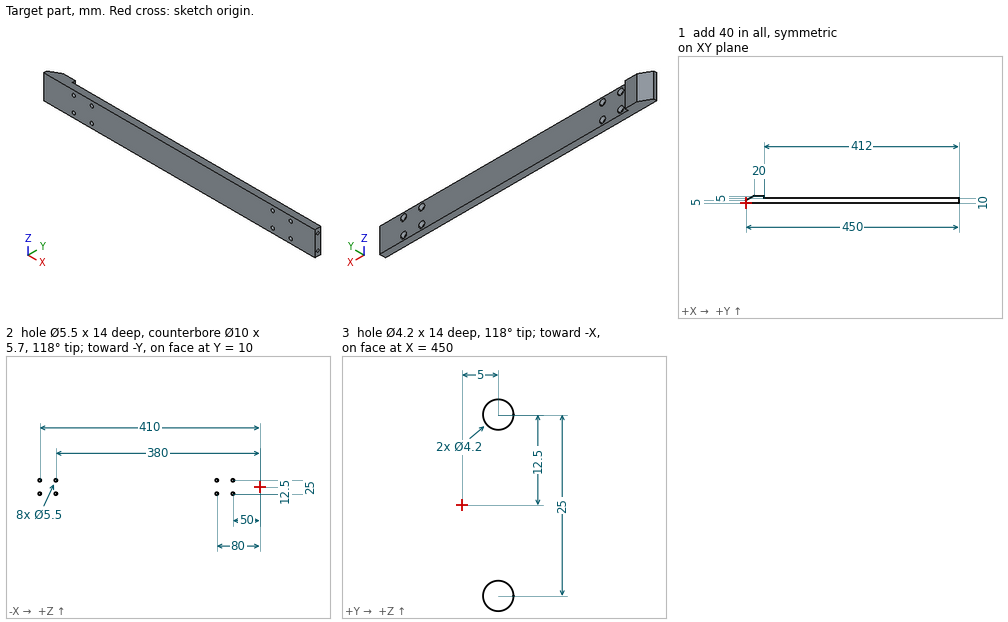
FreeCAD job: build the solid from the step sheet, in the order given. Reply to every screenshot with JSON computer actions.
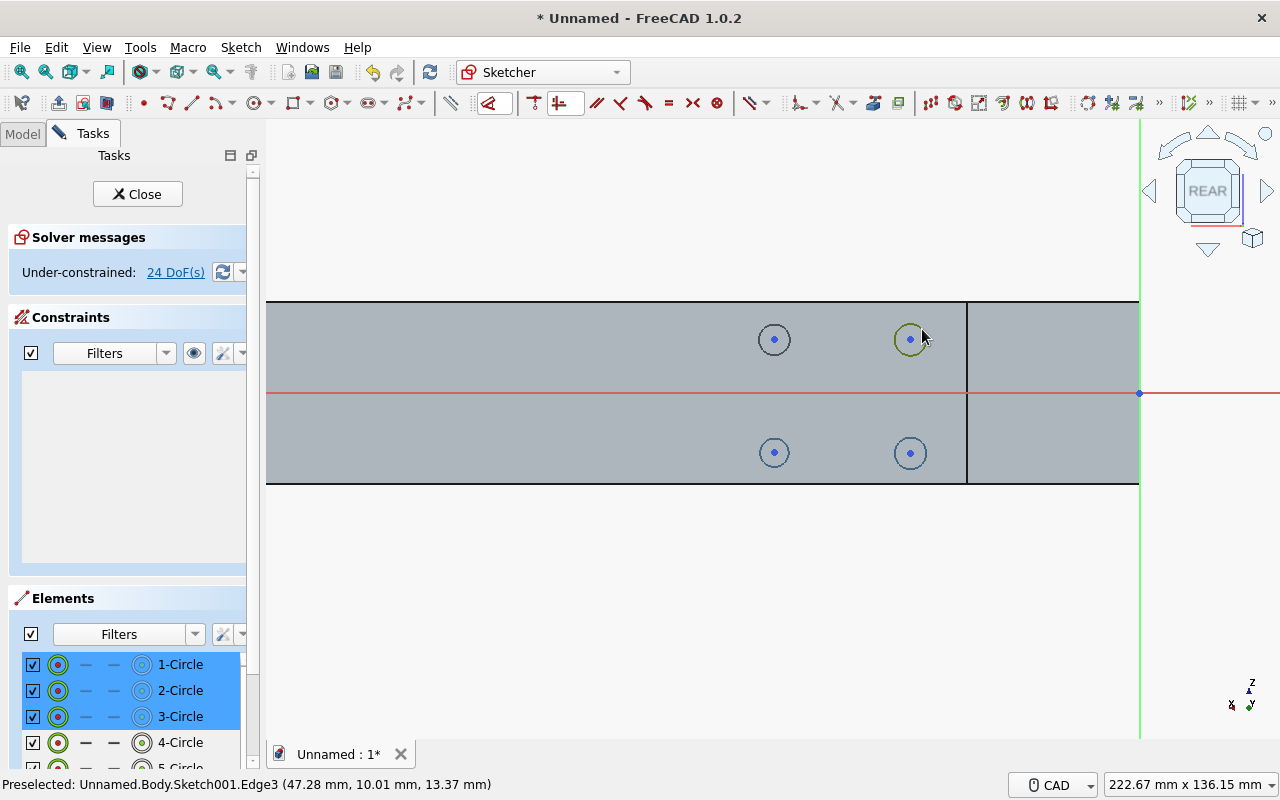
{"action": "left_click", "coordinate": [785, 329]}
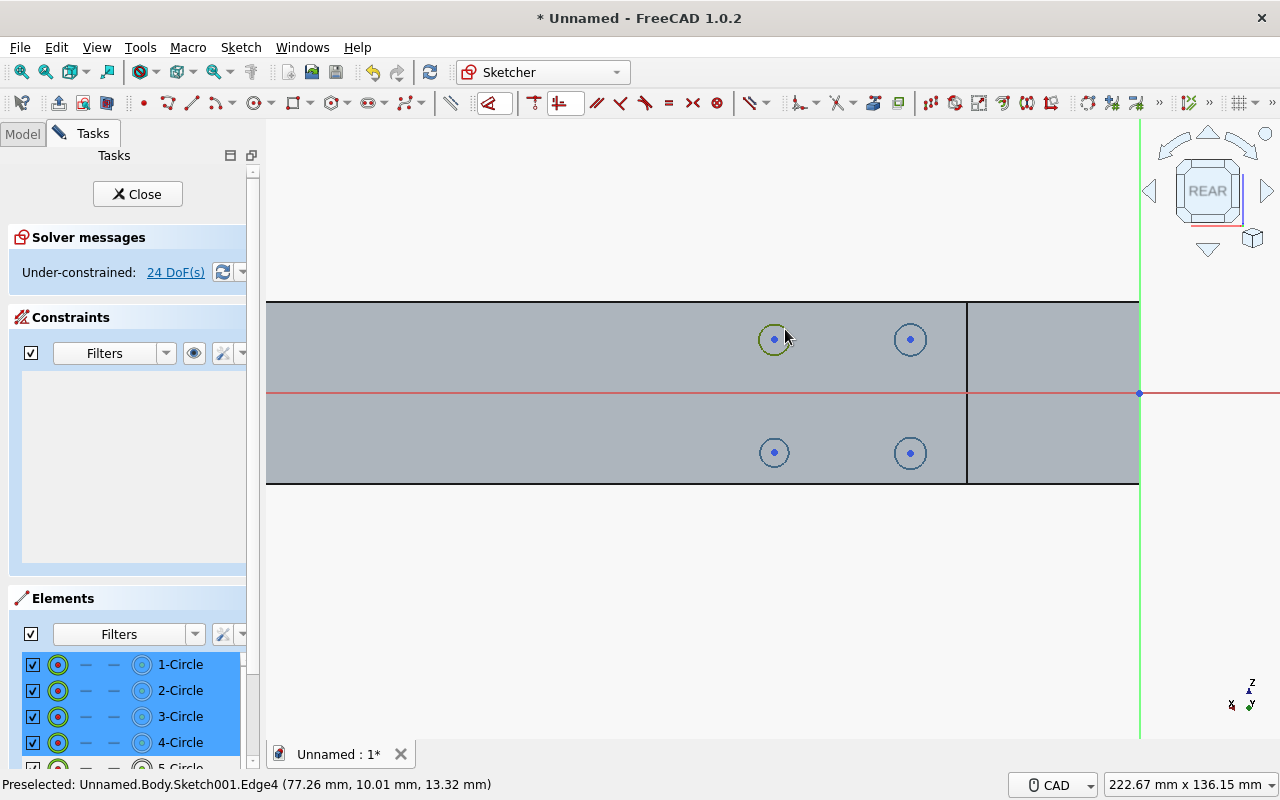
{"action": "scroll", "coordinate": [922, 444], "scroll_direction": "down", "scroll_amount": 6}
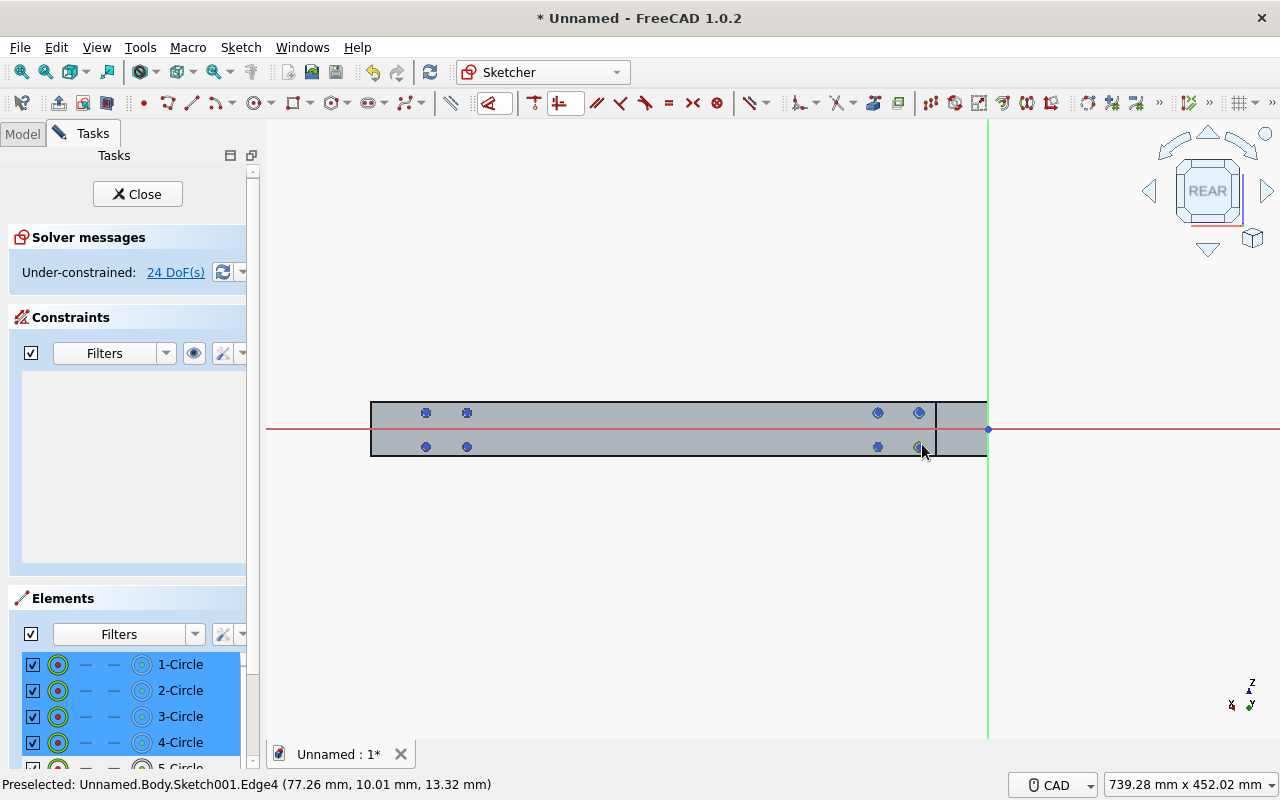
{"action": "scroll", "coordinate": [470, 410], "scroll_direction": "up", "scroll_amount": 6}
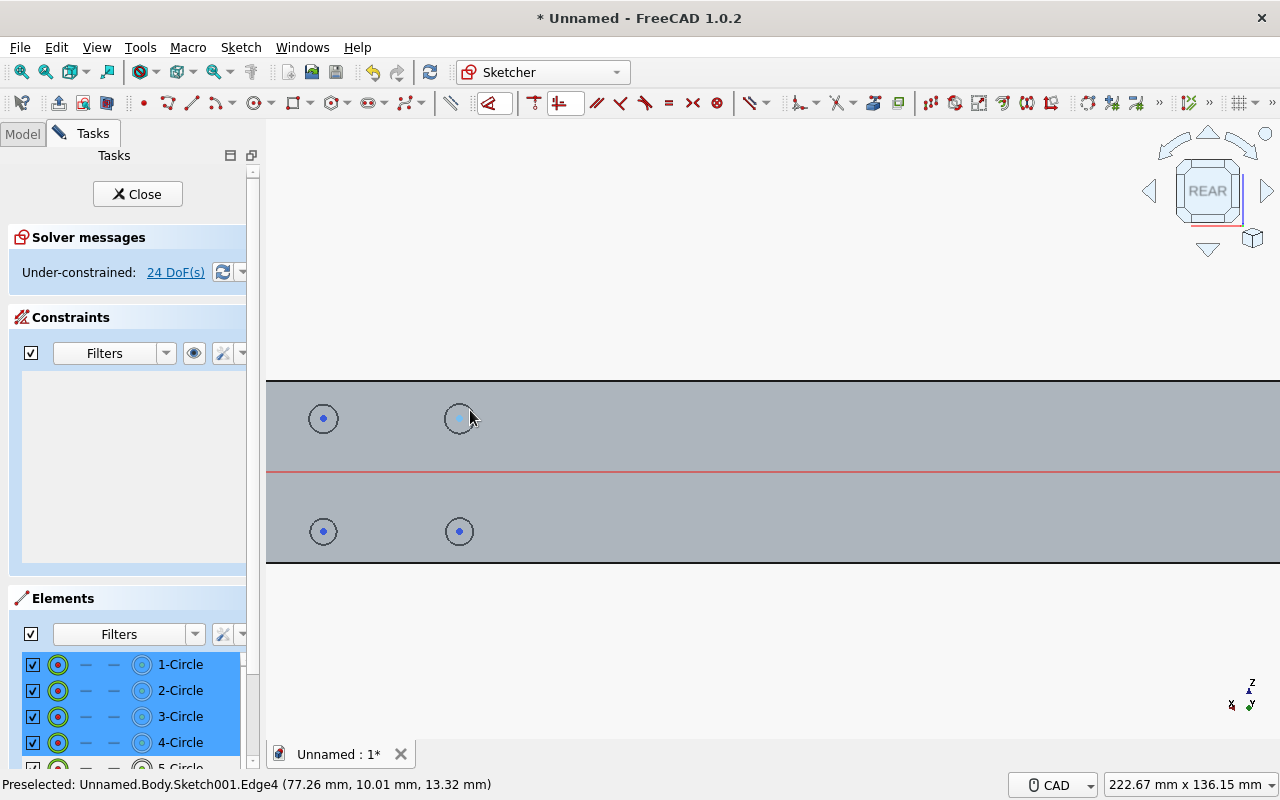
{"action": "left_click", "coordinate": [470, 408]}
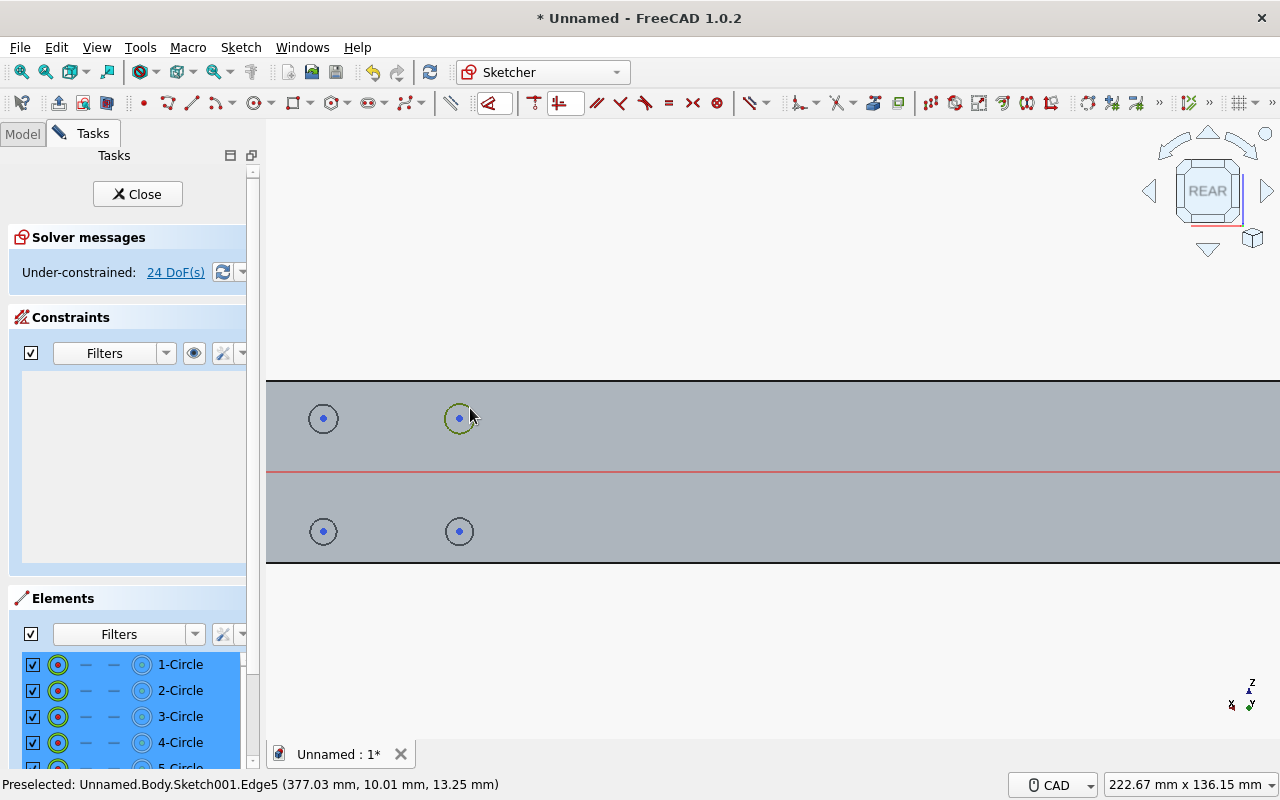
{"action": "left_click", "coordinate": [334, 409]}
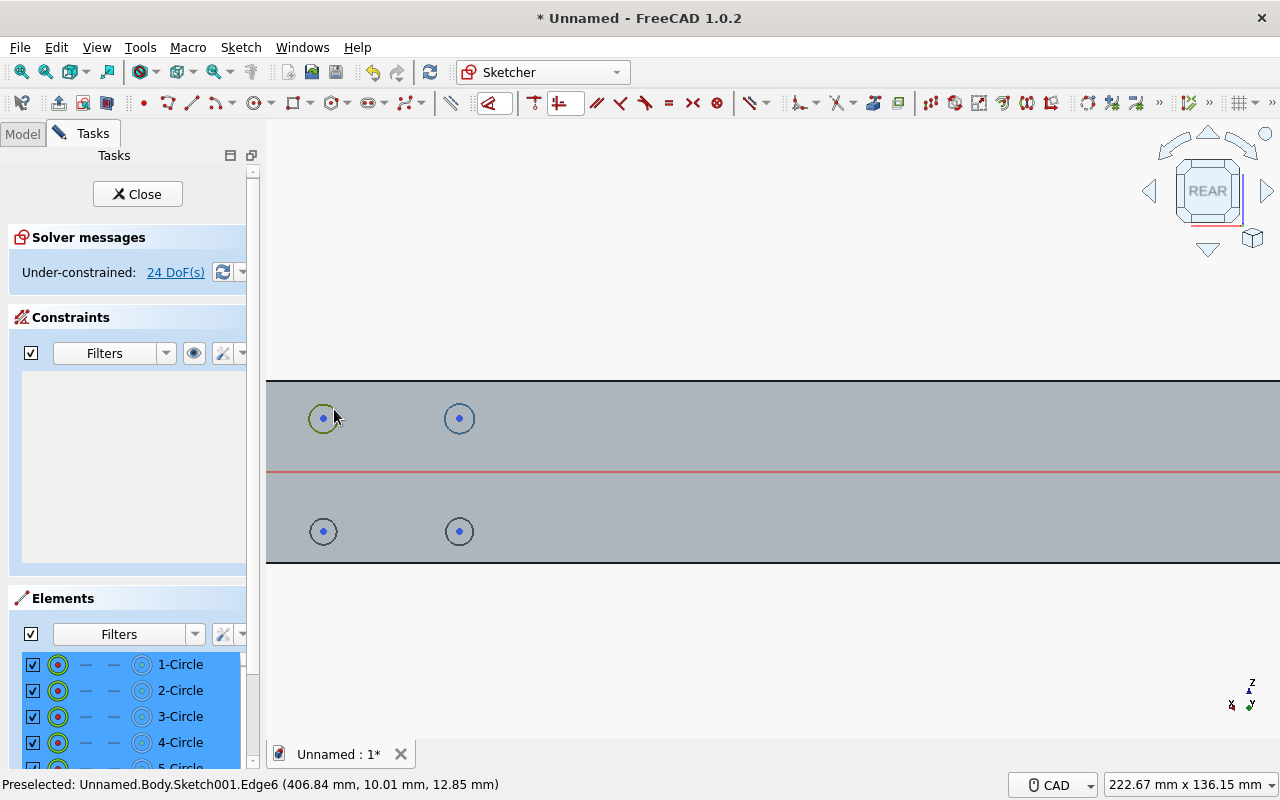
{"action": "left_click", "coordinate": [469, 522]}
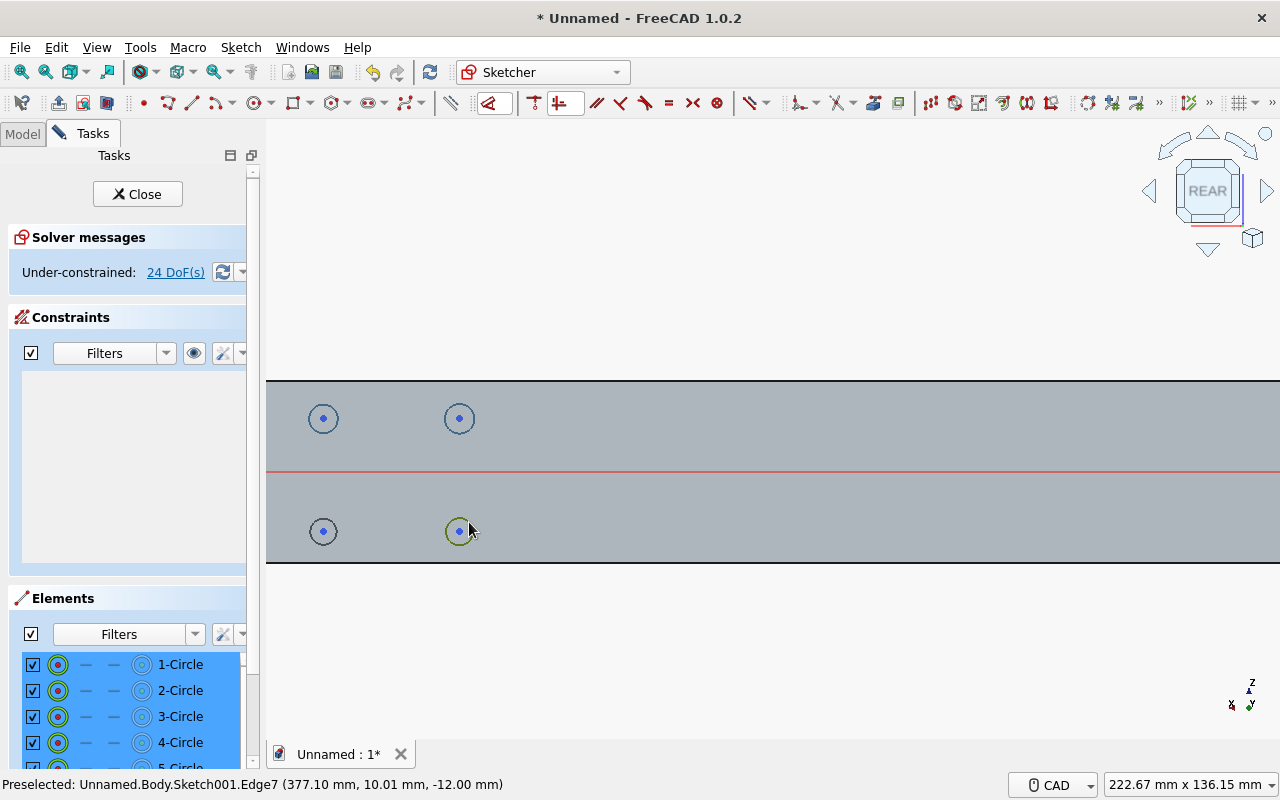
{"action": "left_click", "coordinate": [333, 522]}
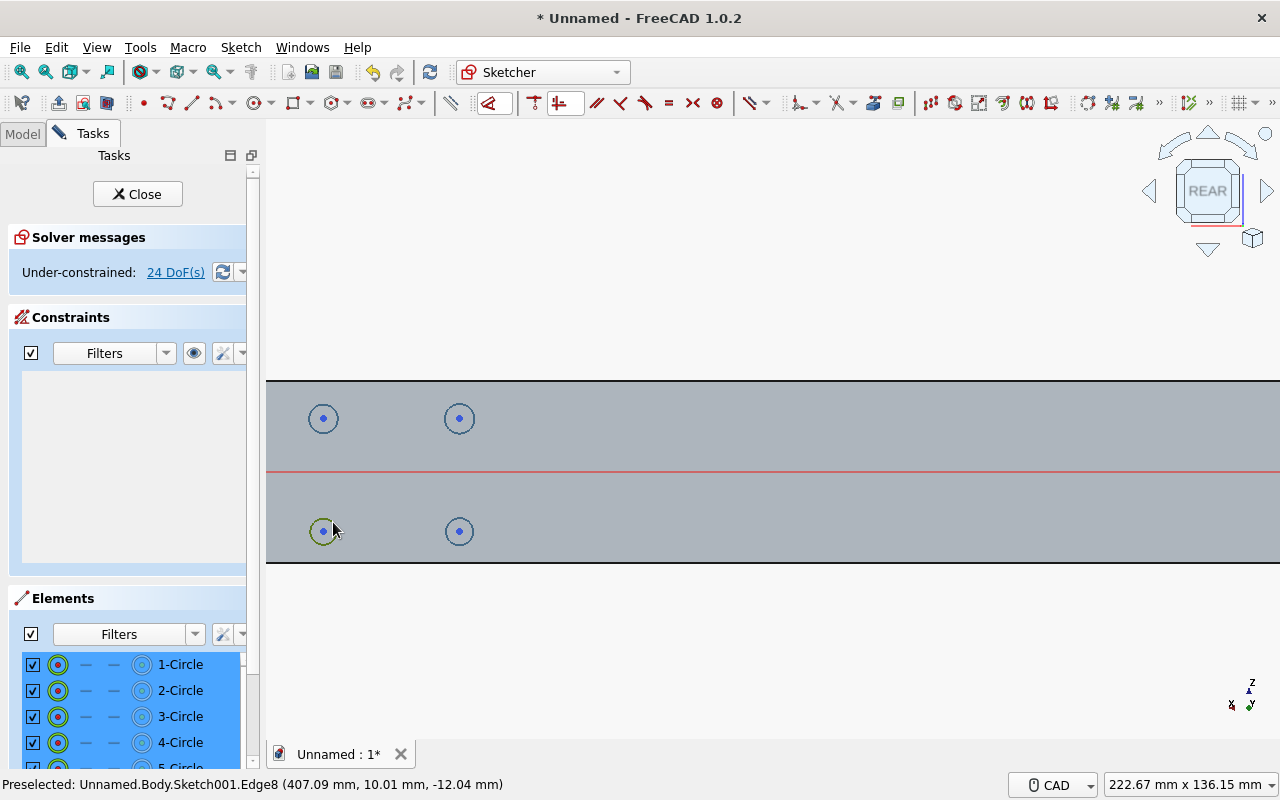
{"action": "left_click", "coordinate": [670, 104]}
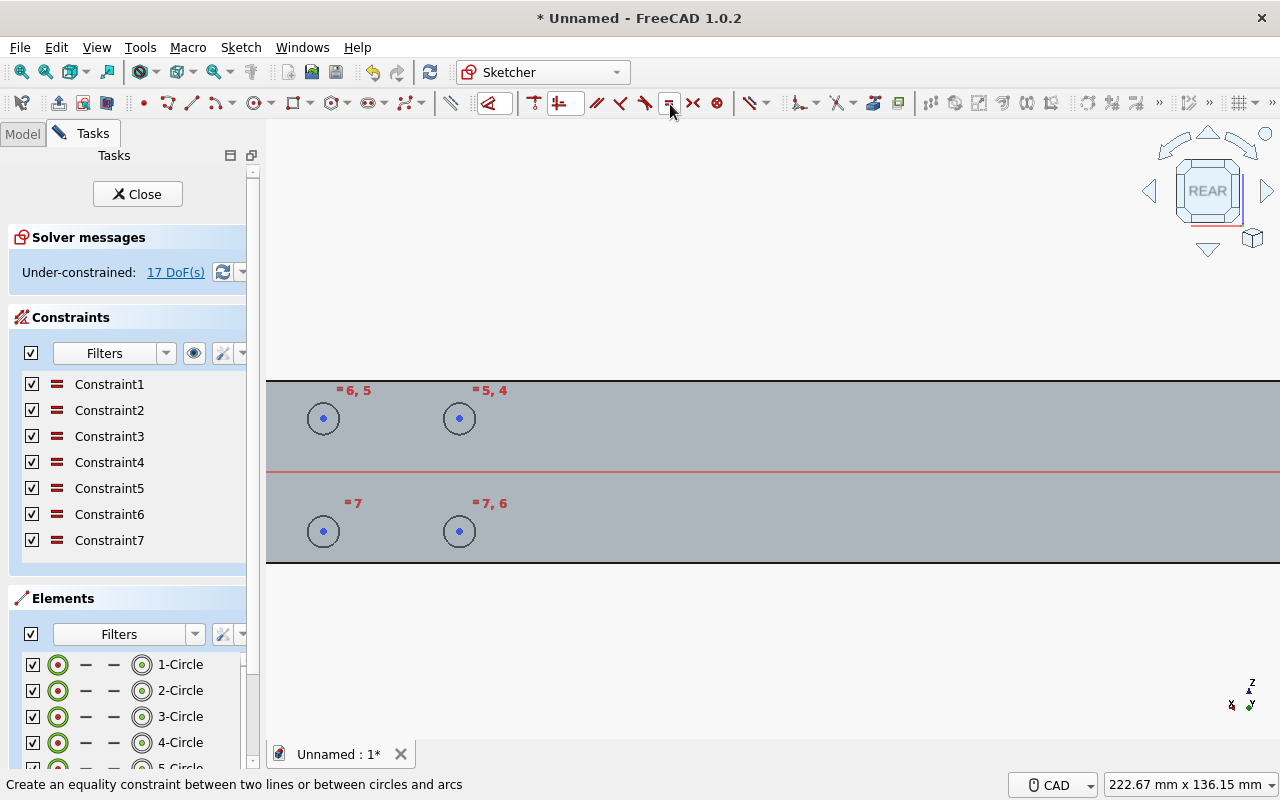
{"action": "scroll", "coordinate": [470, 410], "scroll_direction": "down", "scroll_amount": 6}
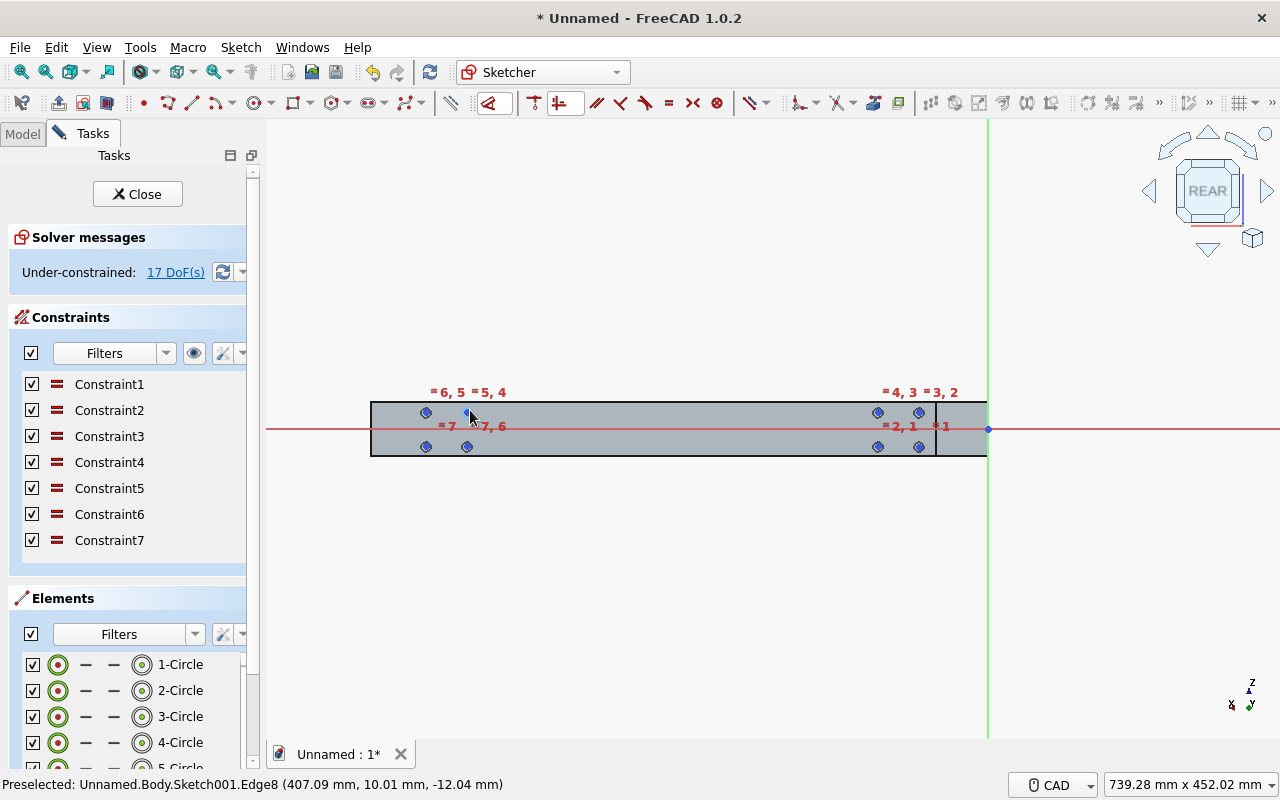
{"action": "left_click", "coordinate": [919, 447]}